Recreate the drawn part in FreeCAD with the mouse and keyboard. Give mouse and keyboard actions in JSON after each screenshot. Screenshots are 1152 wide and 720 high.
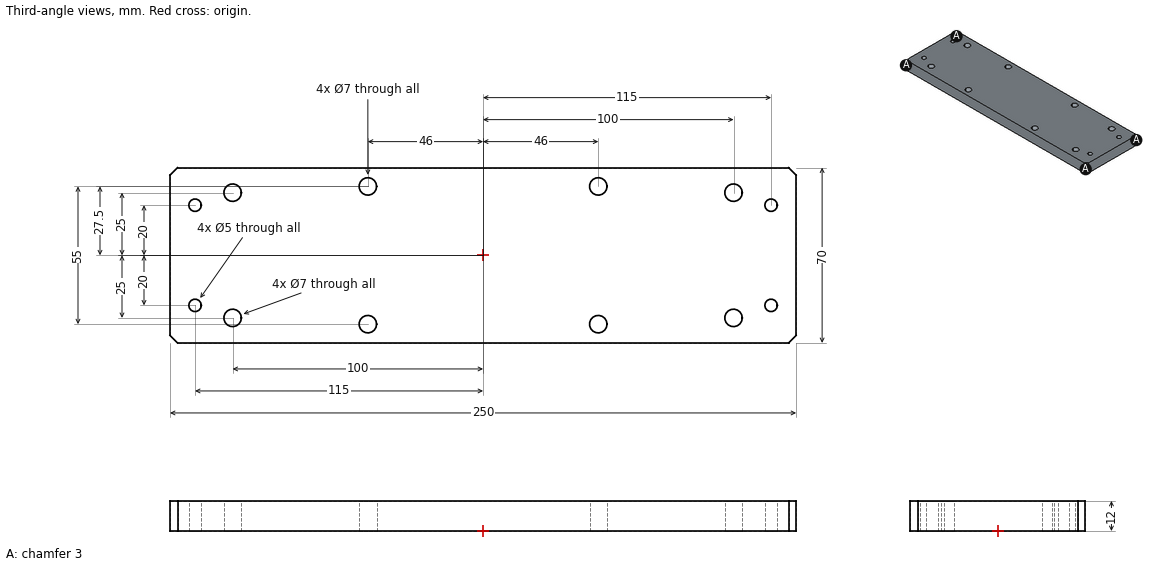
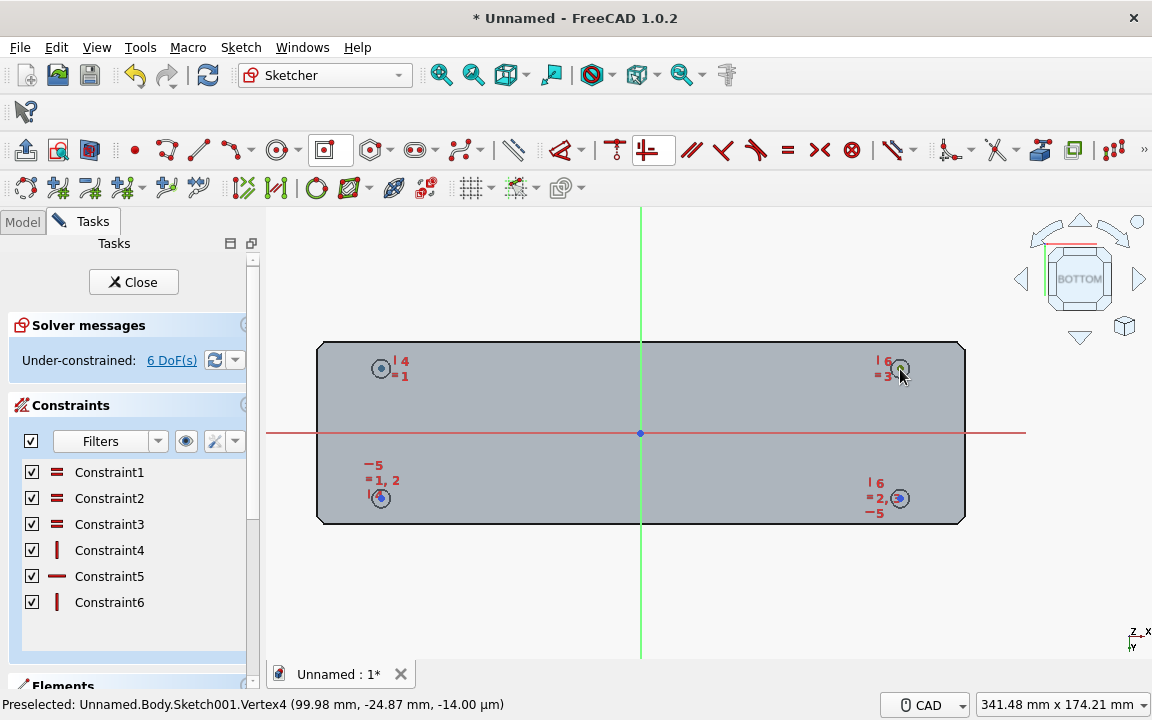
{"action": "left_click", "coordinate": [670, 150]}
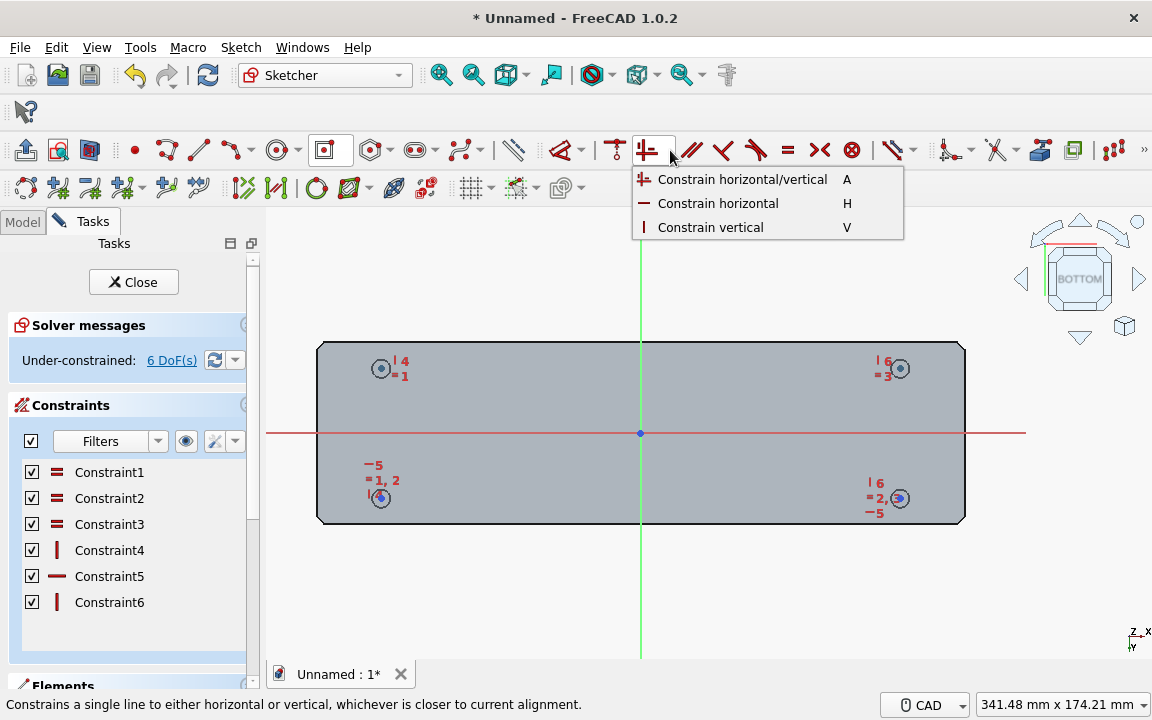
{"action": "left_click", "coordinate": [768, 203]}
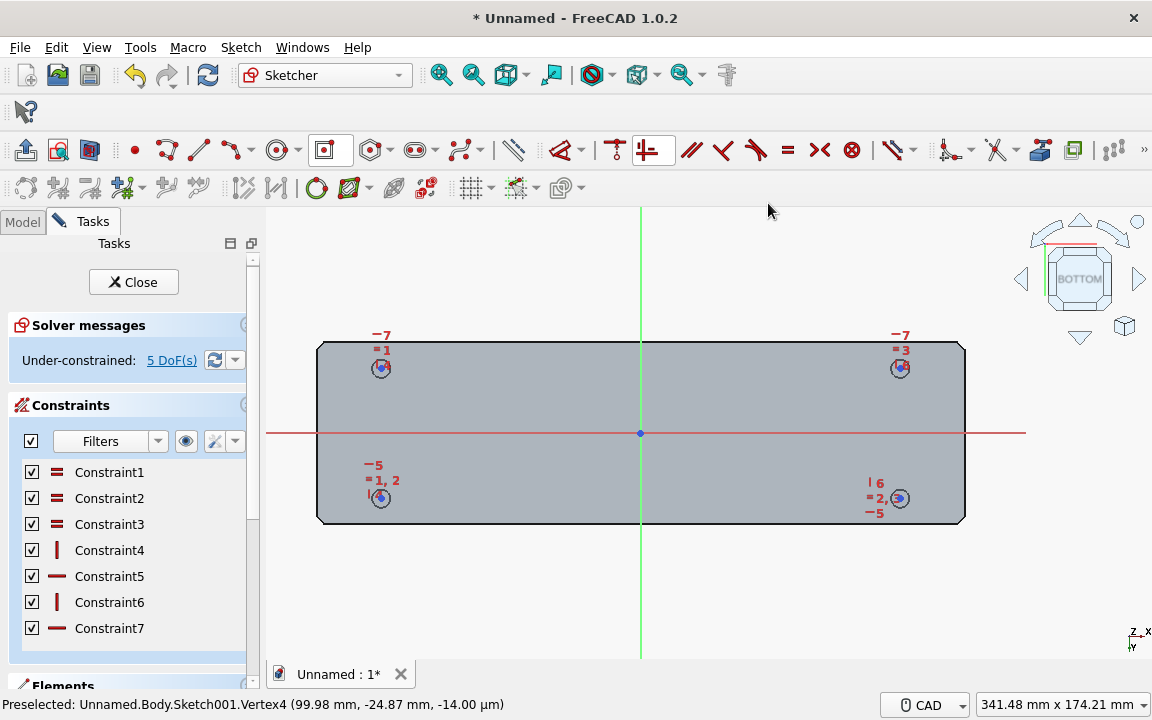
{"action": "scroll", "coordinate": [388, 362], "scroll_direction": "up", "scroll_amount": 4}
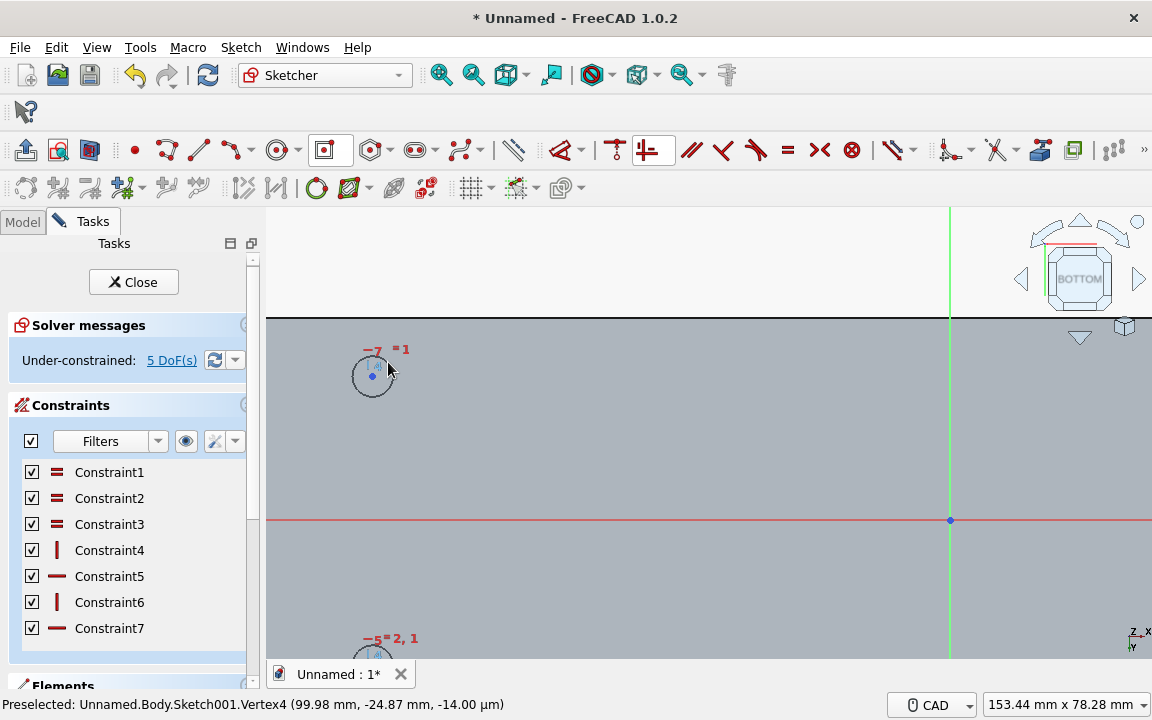
{"action": "left_click", "coordinate": [387, 362]}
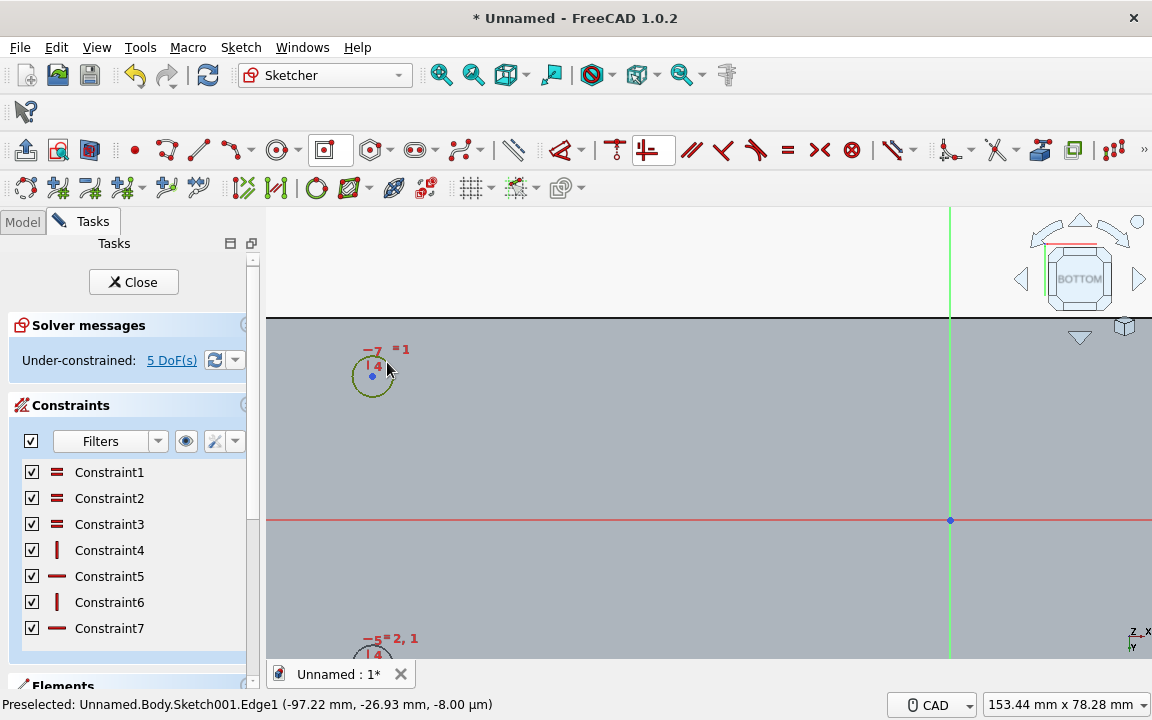
{"action": "key", "text": "k o"}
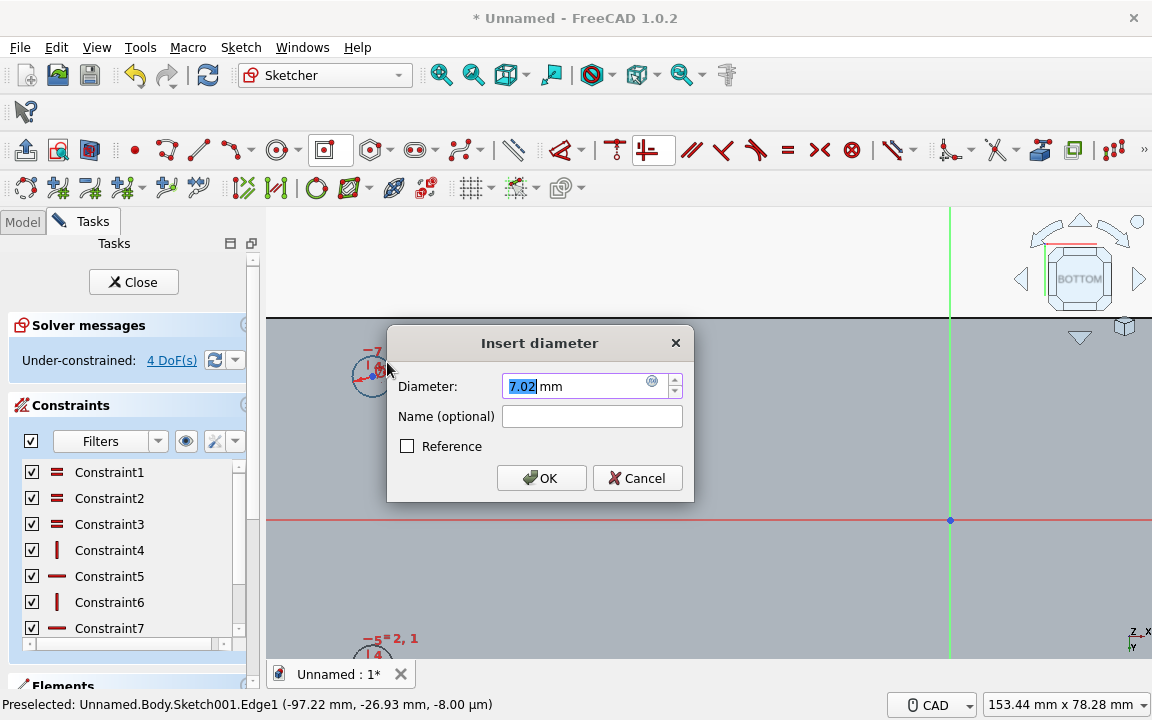
{"action": "type", "text": "7"}
{"action": "key", "text": "Return"}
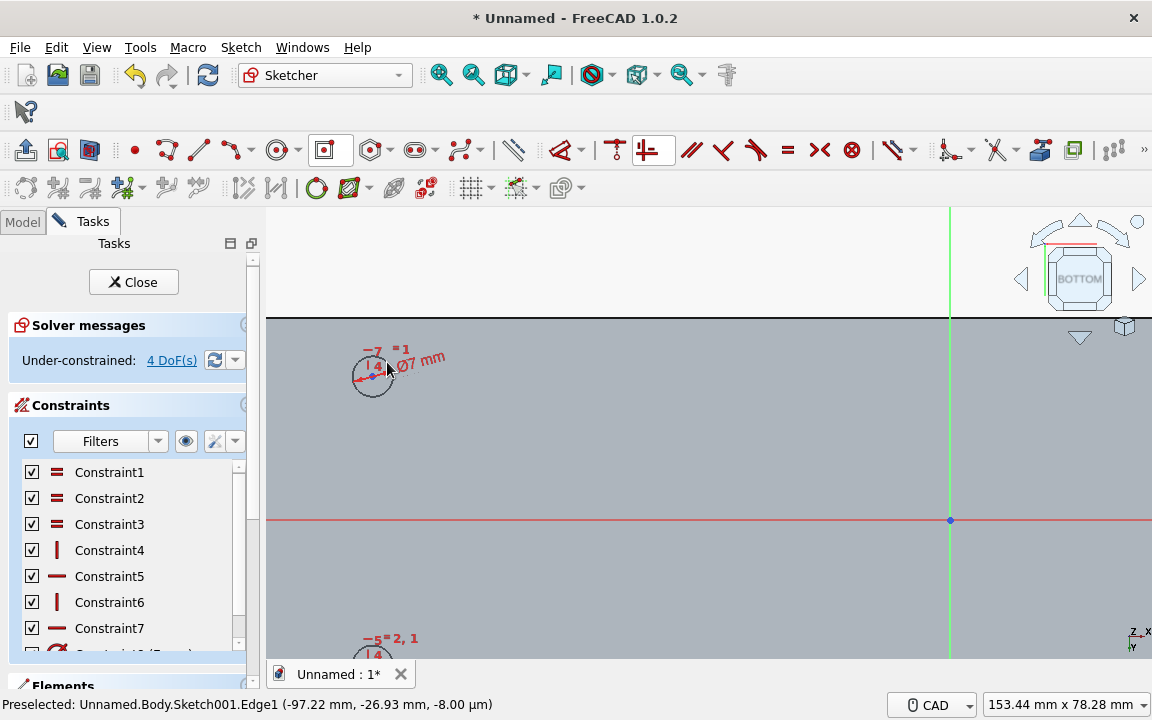
{"action": "left_click", "coordinate": [373, 377]}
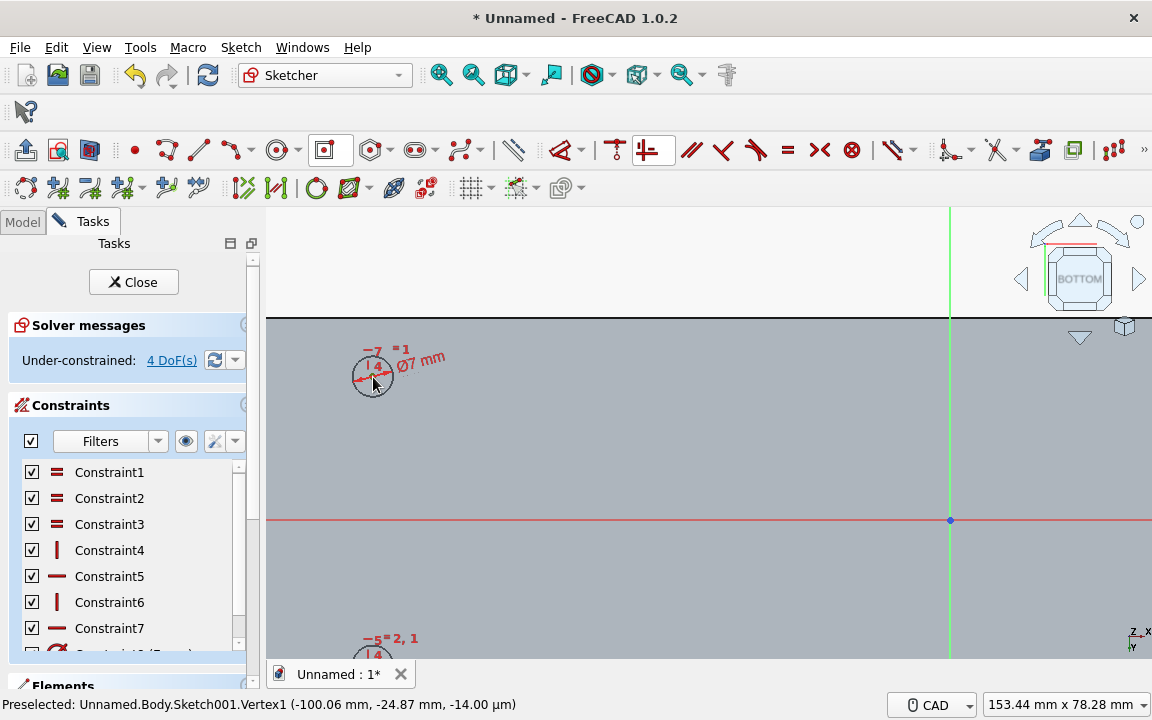
{"action": "key", "text": "i"}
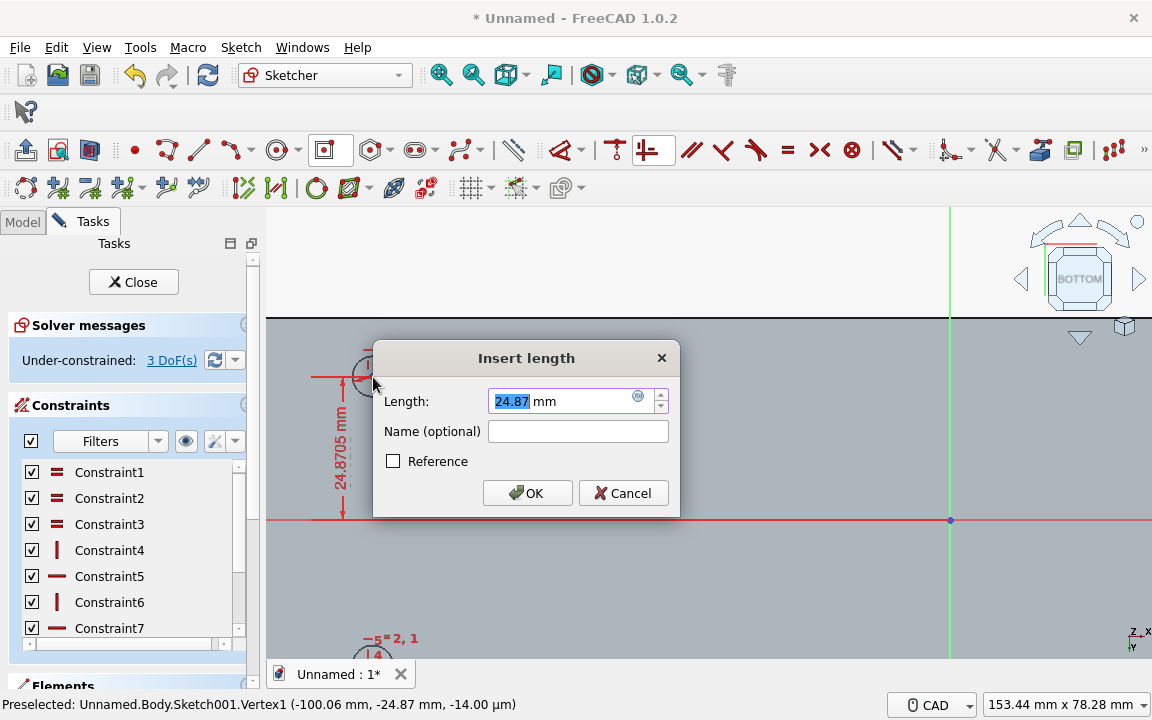
{"action": "type", "text": "25"}
{"action": "key", "text": "Return"}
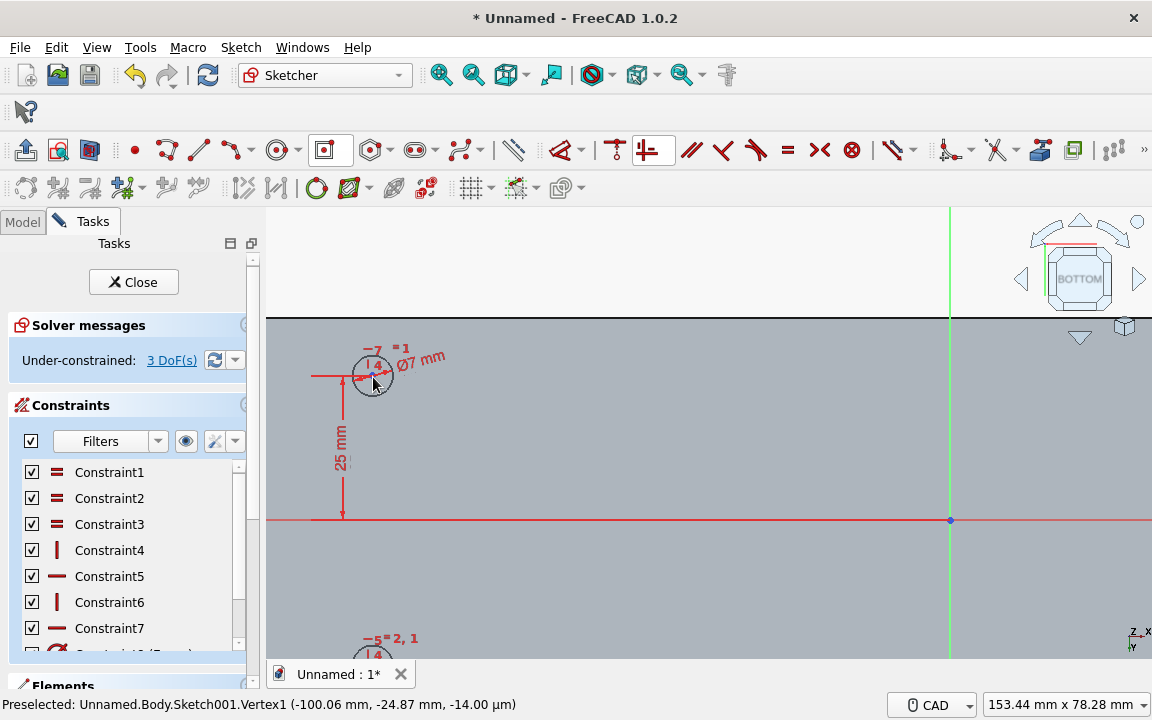
{"action": "scroll", "coordinate": [388, 362], "scroll_direction": "down", "scroll_amount": 4}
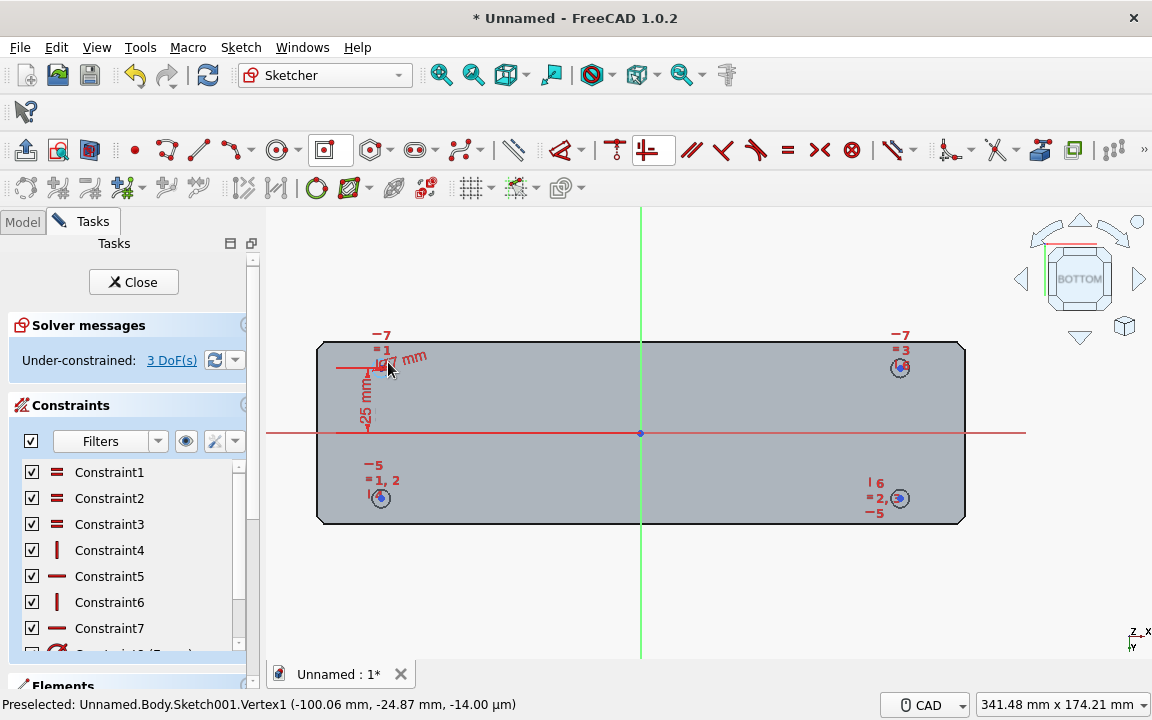
{"action": "left_click", "coordinate": [381, 499]}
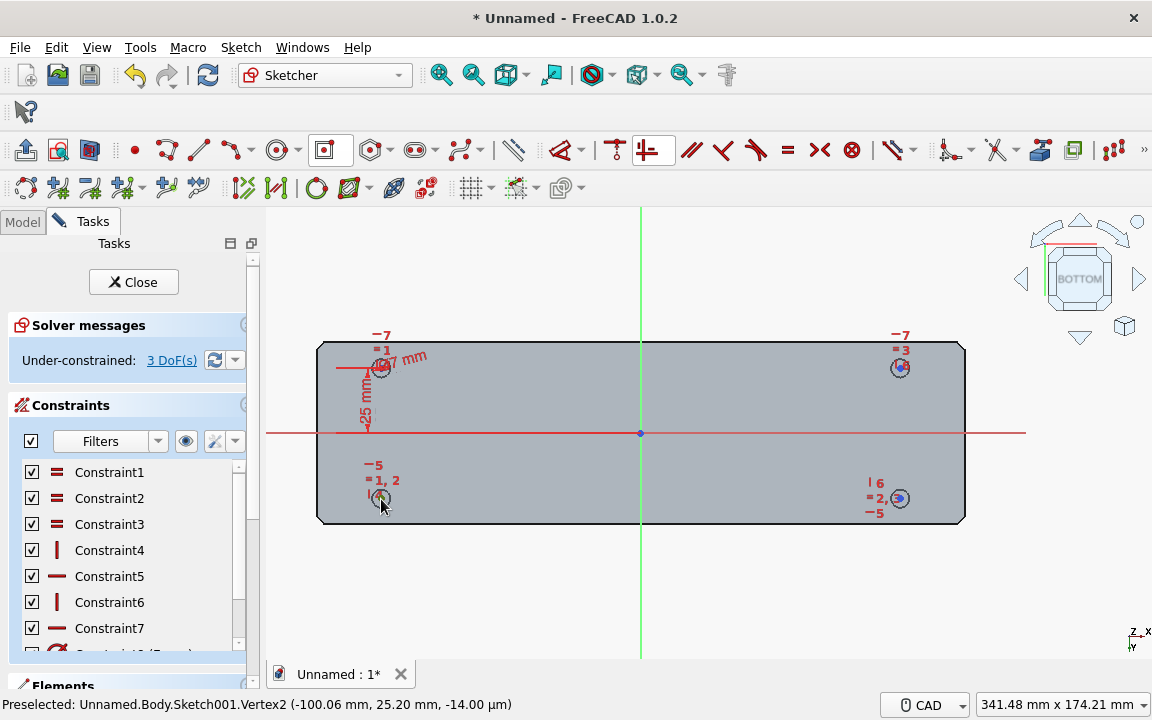
{"action": "left_click", "coordinate": [584, 150]}